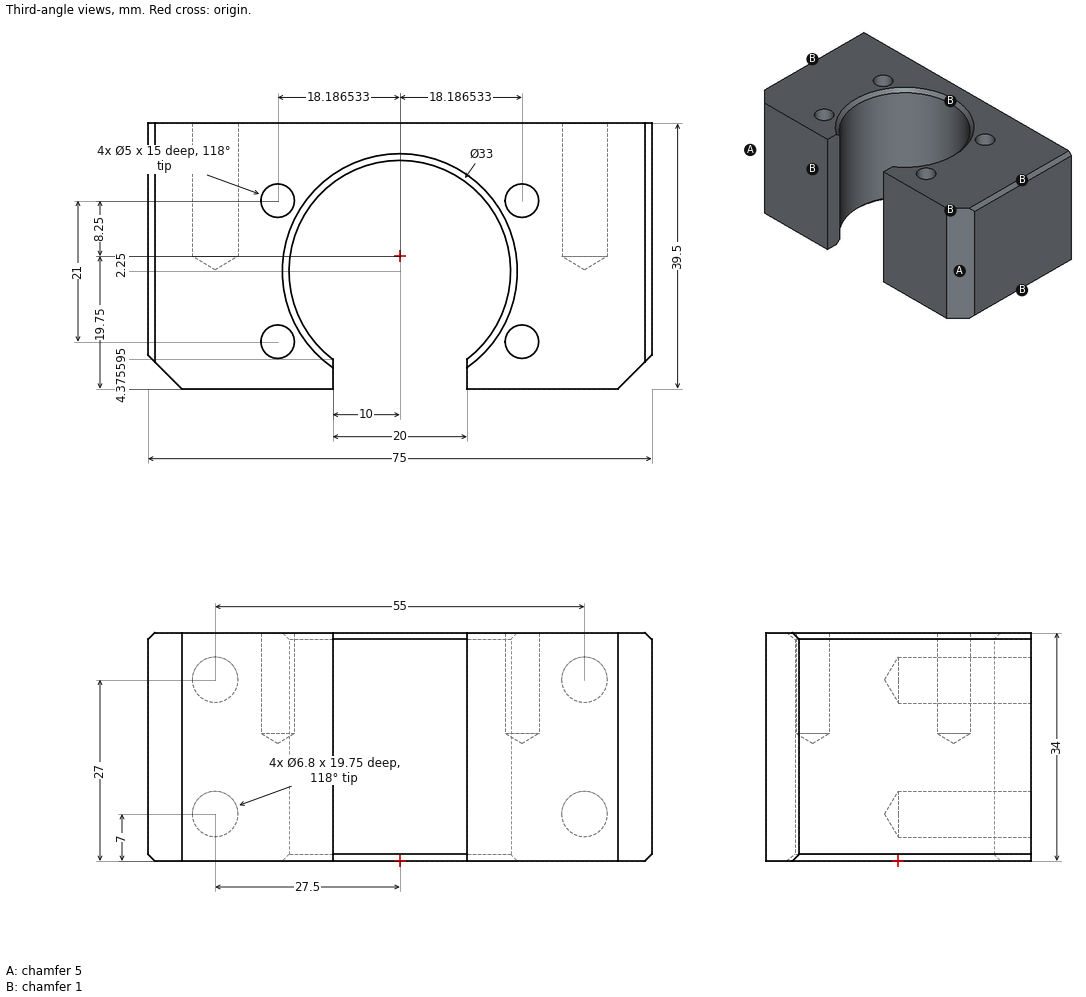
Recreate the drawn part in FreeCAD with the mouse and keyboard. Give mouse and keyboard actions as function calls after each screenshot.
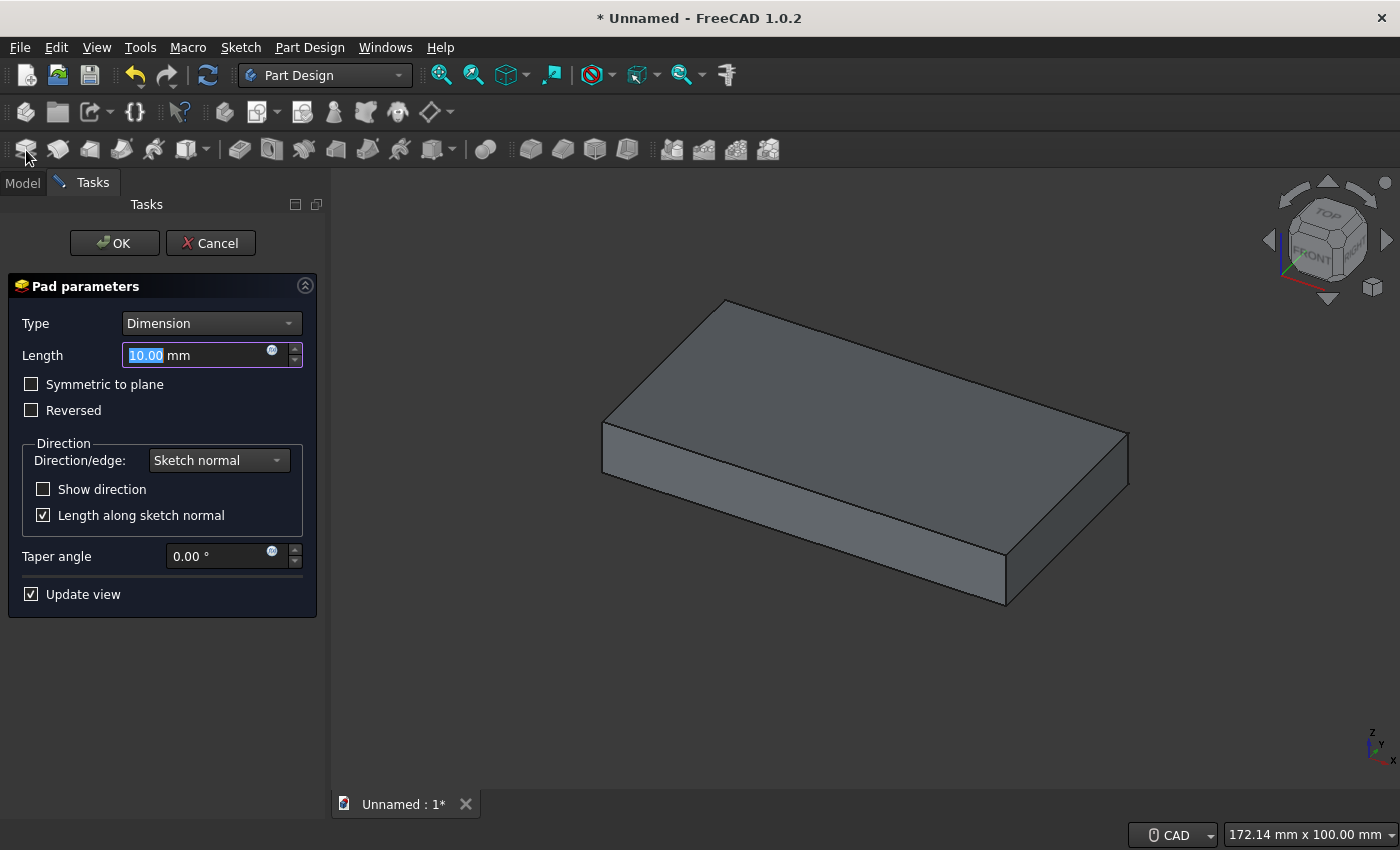
text(34)
key(Tab)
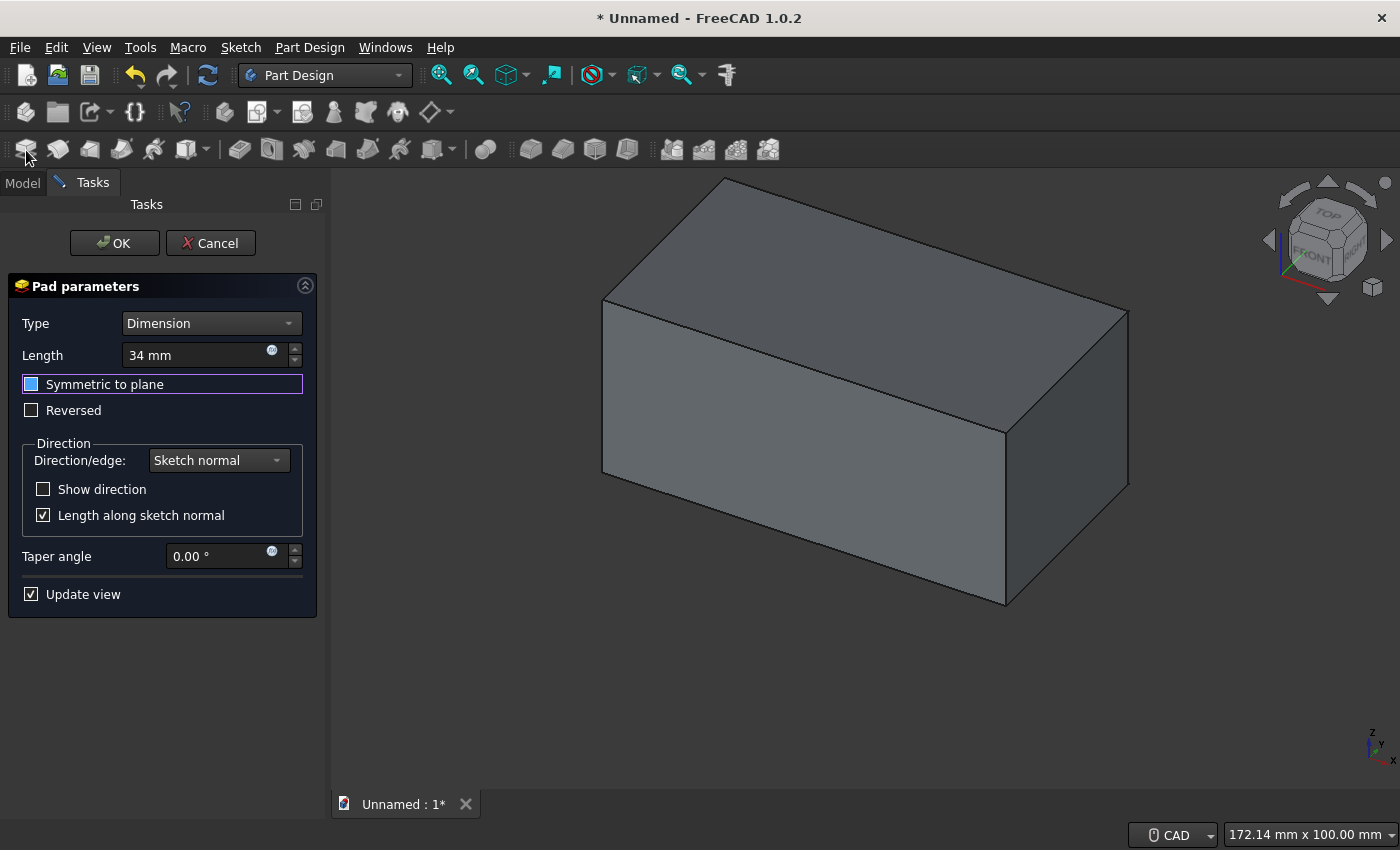
click(115, 243)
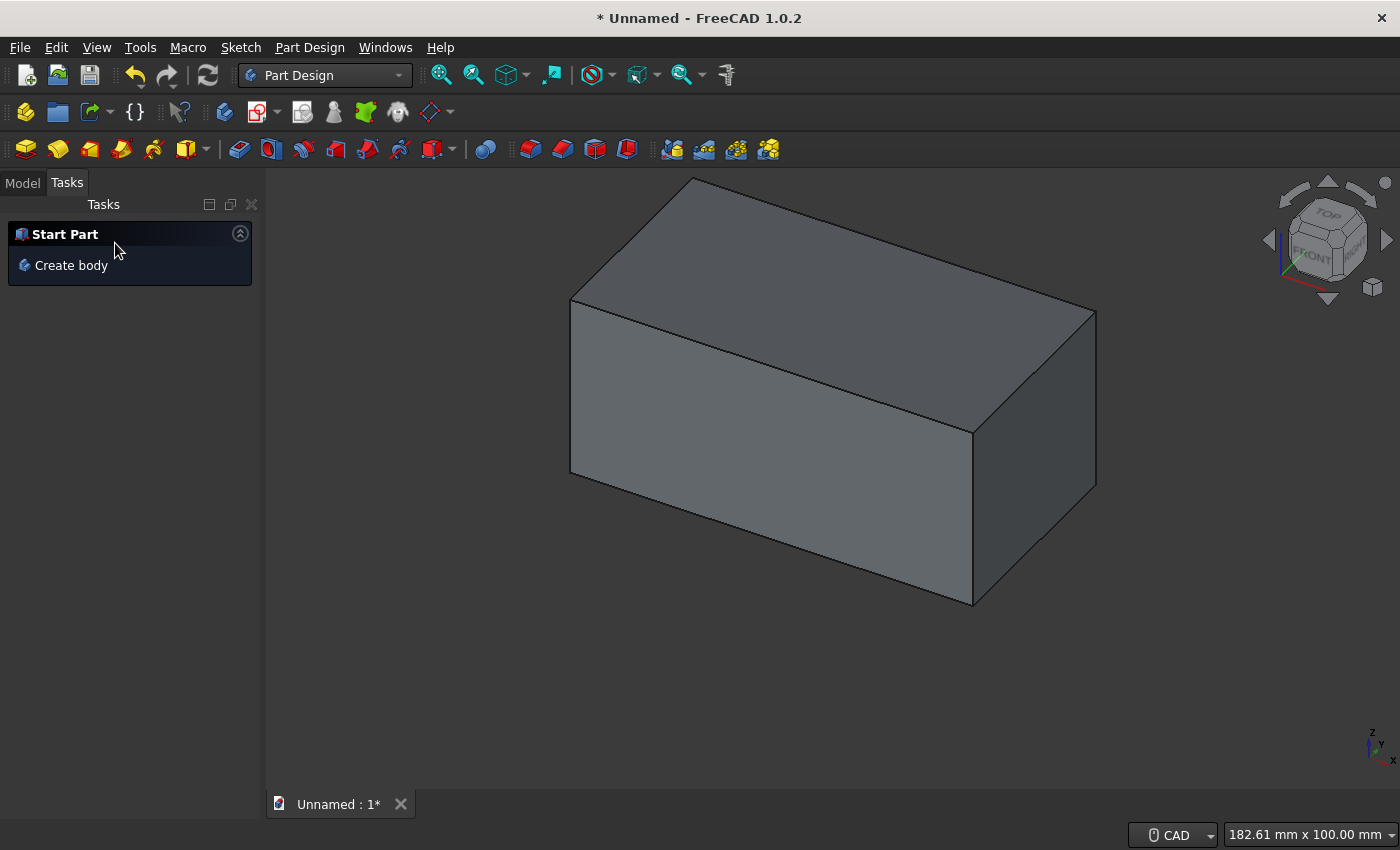
click(891, 324)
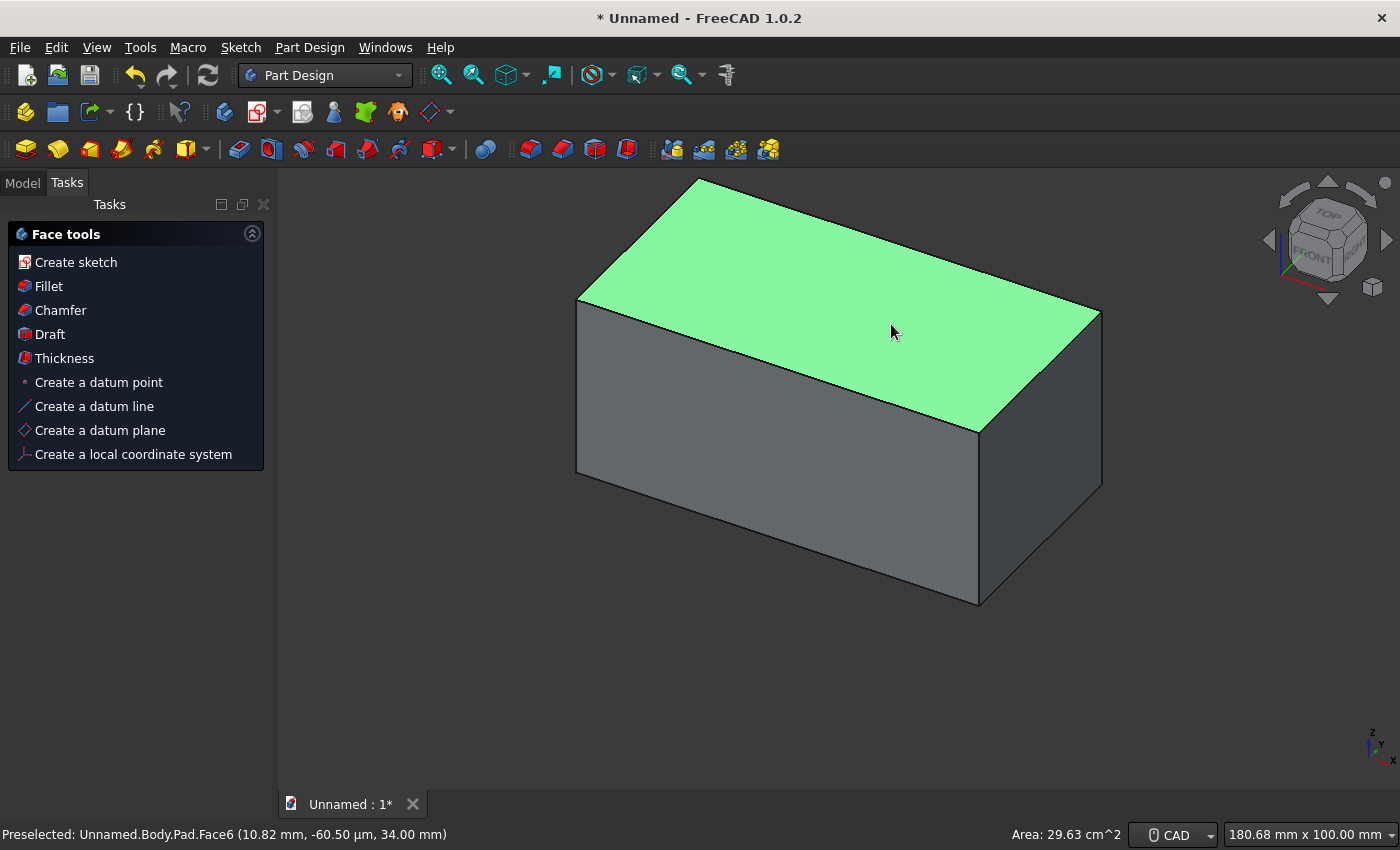
click(258, 112)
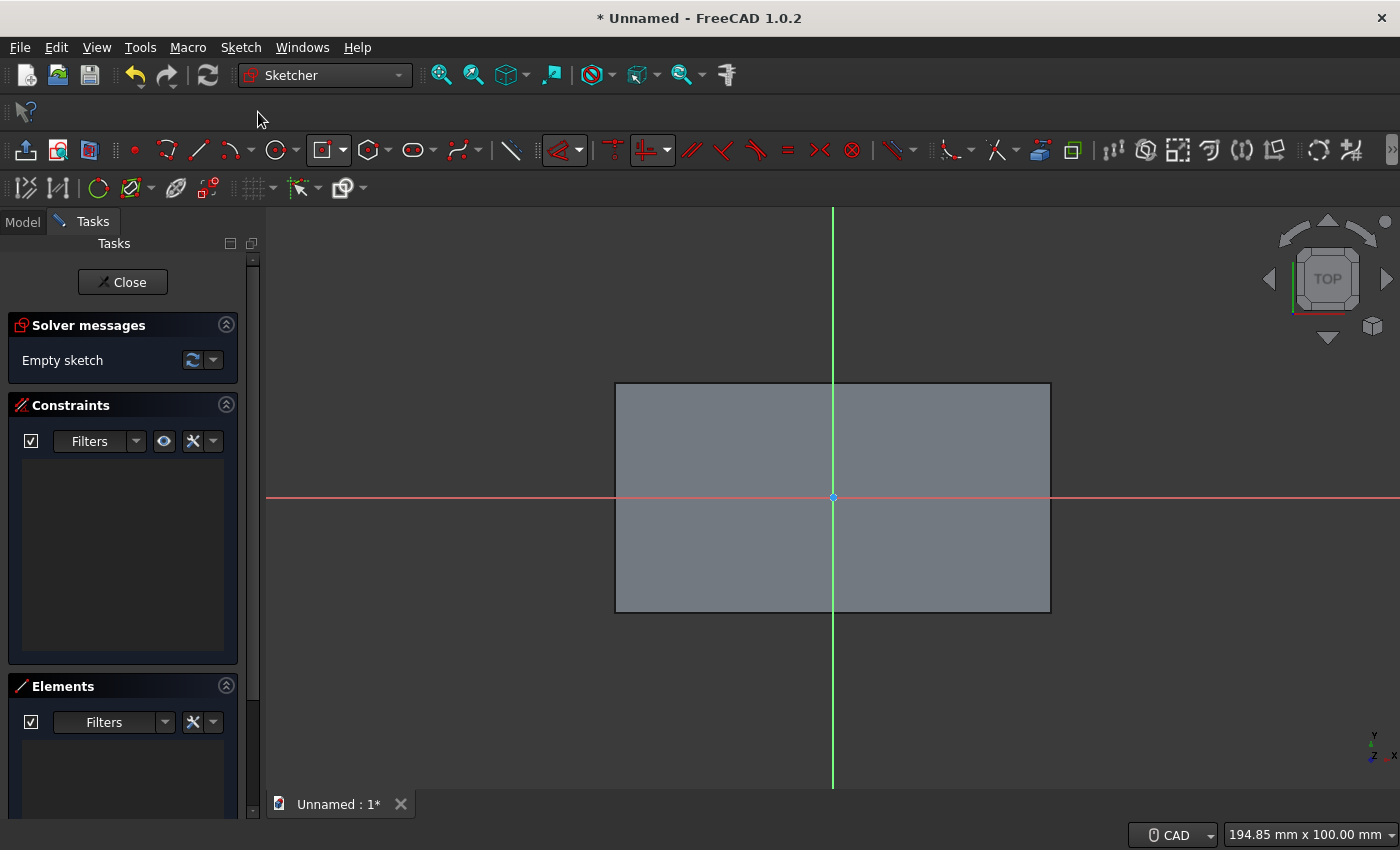
scroll(916, 527, up, 3)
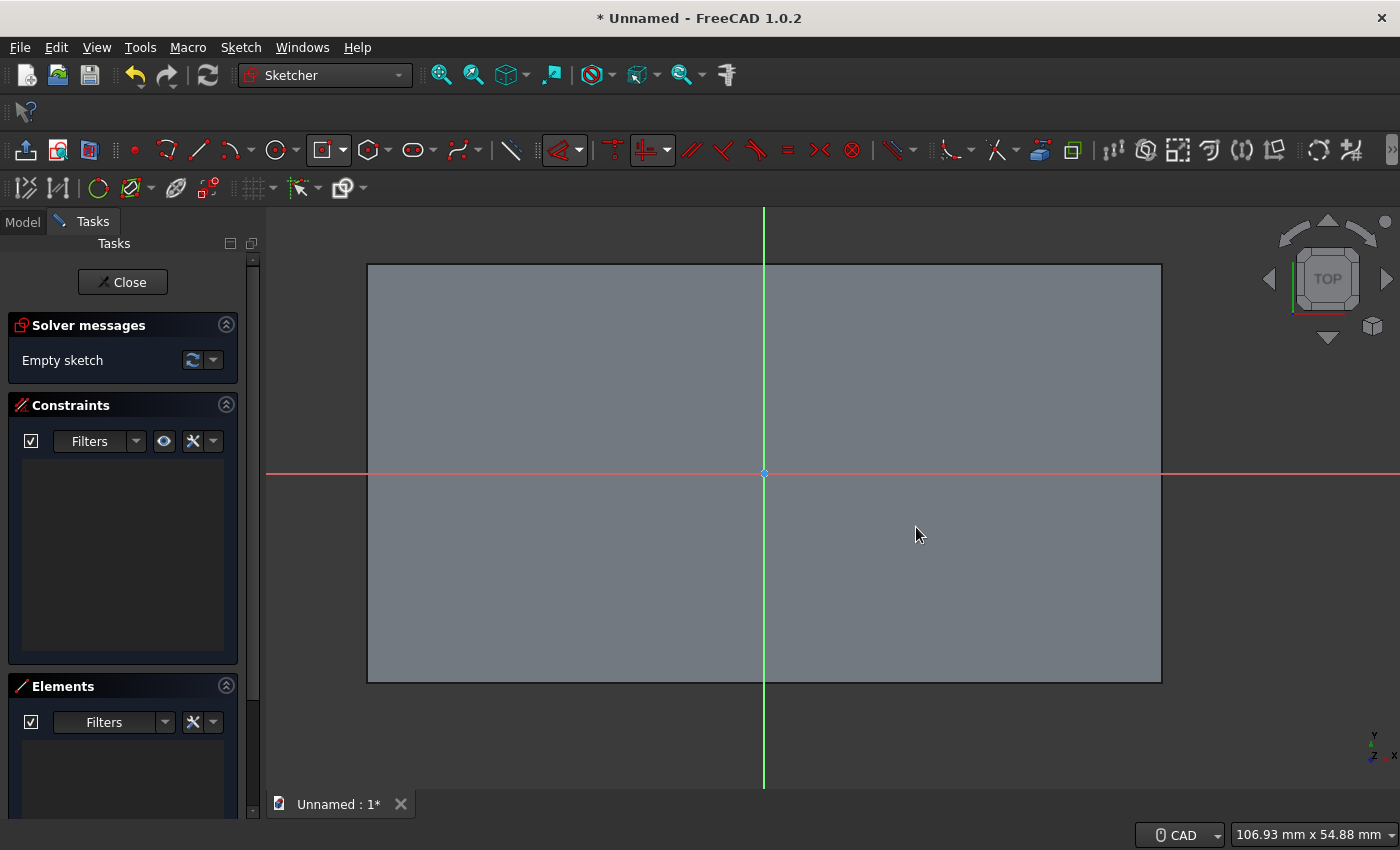
click(276, 150)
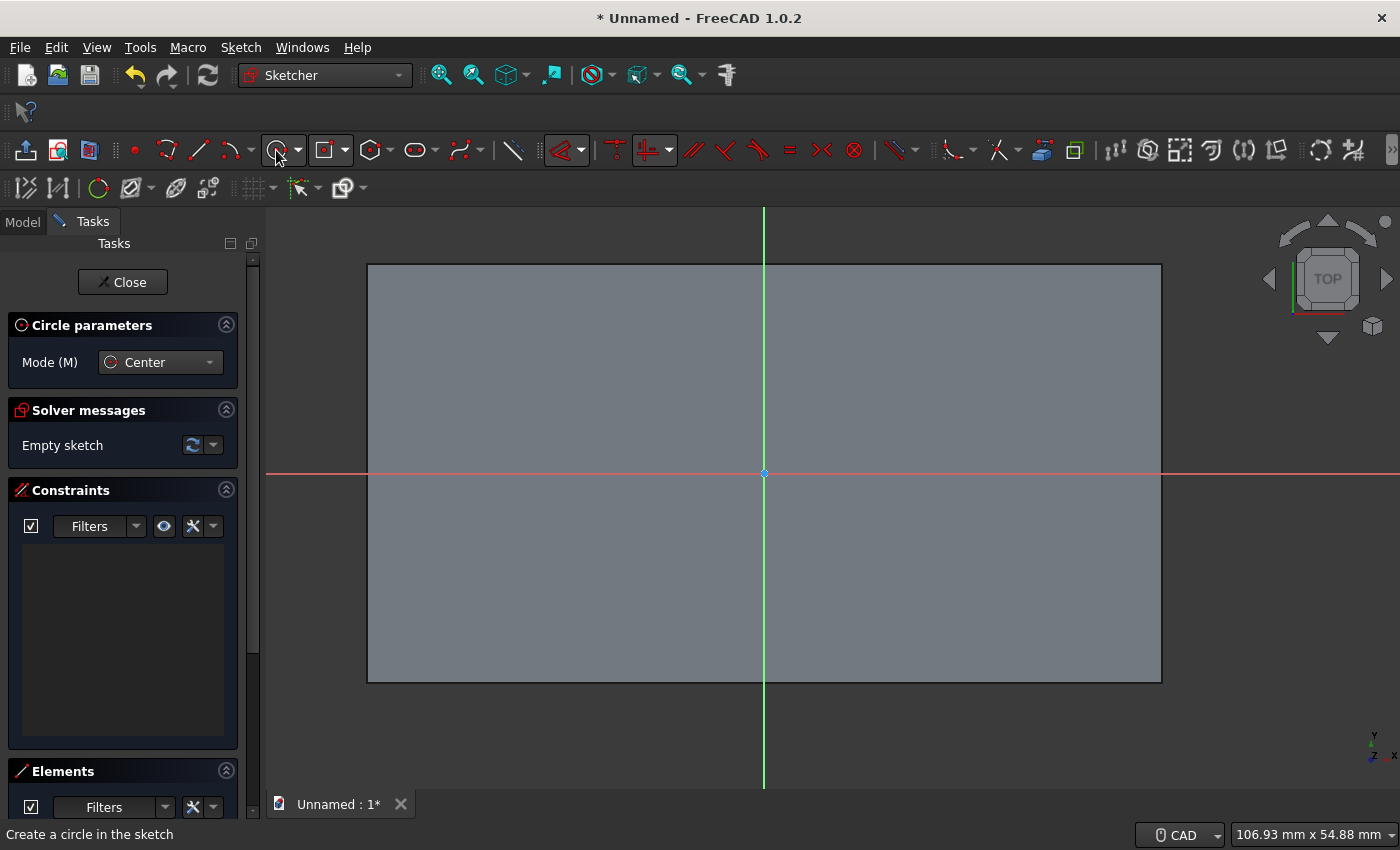
click(764, 498)
click(888, 374)
key(Escape)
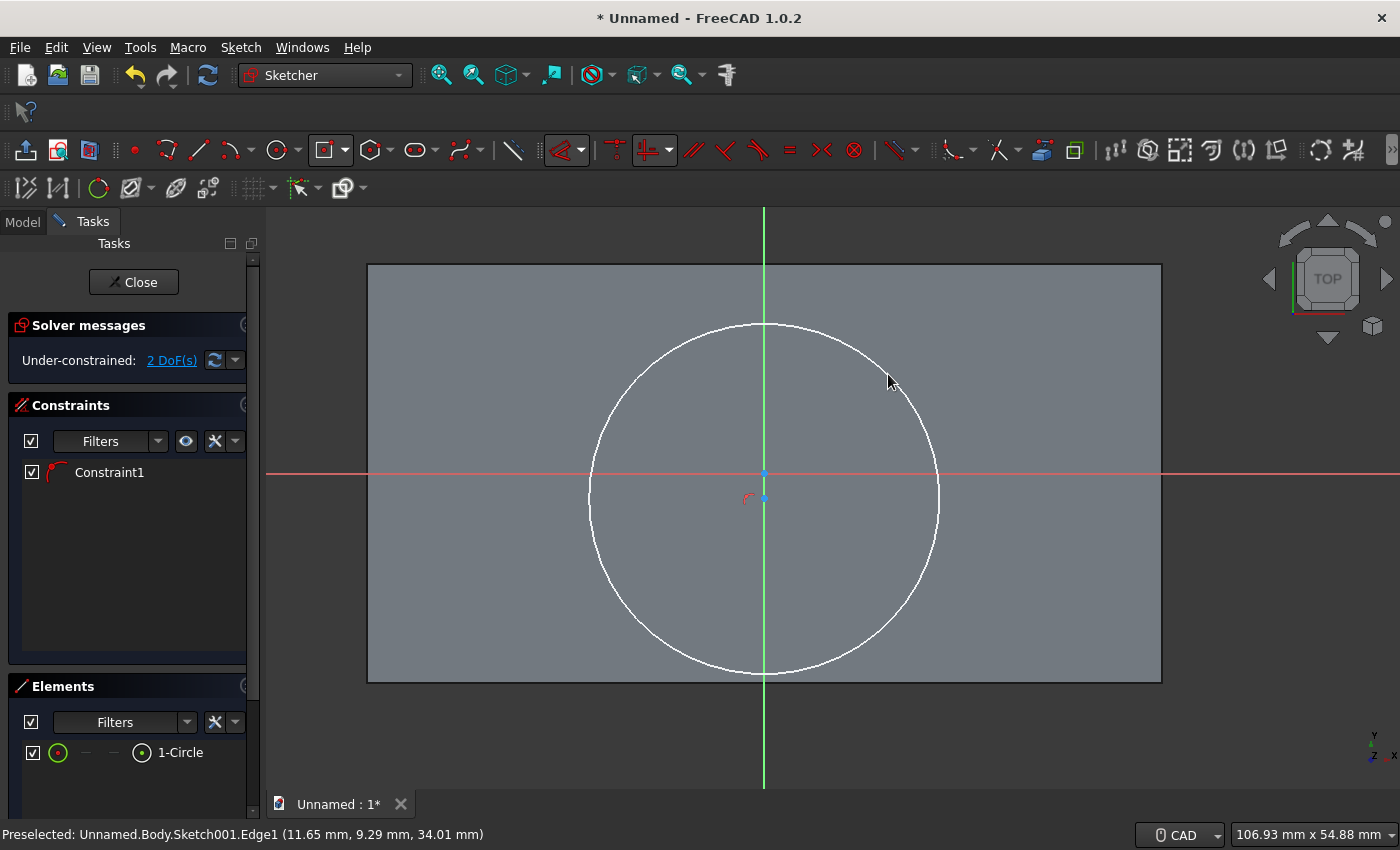
click(888, 375)